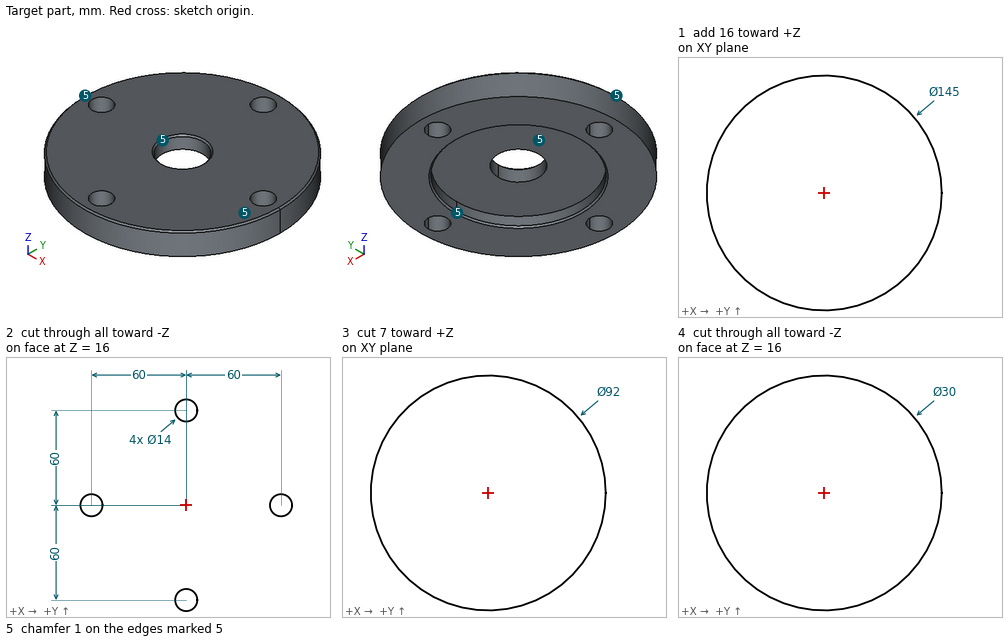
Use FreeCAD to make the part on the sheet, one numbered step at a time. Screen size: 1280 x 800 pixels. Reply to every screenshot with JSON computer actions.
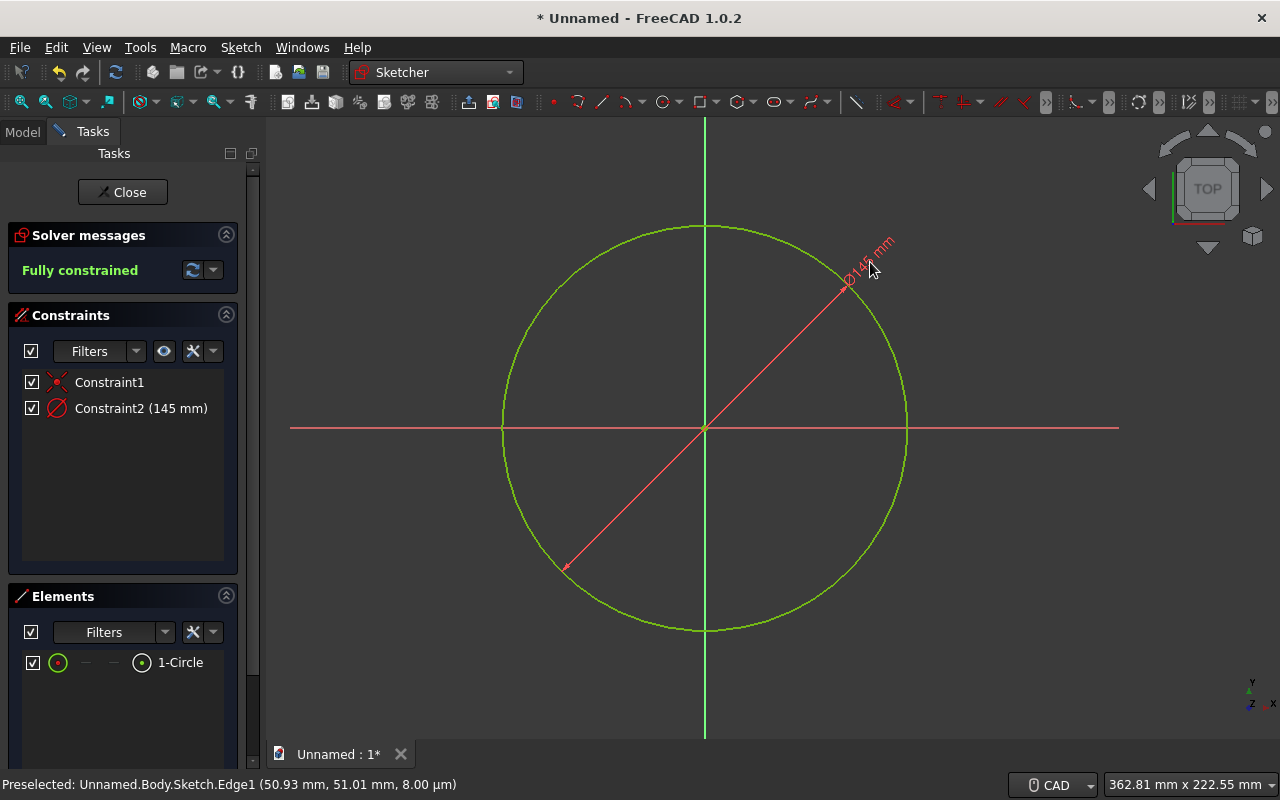
{"action": "left_click", "coordinate": [123, 192]}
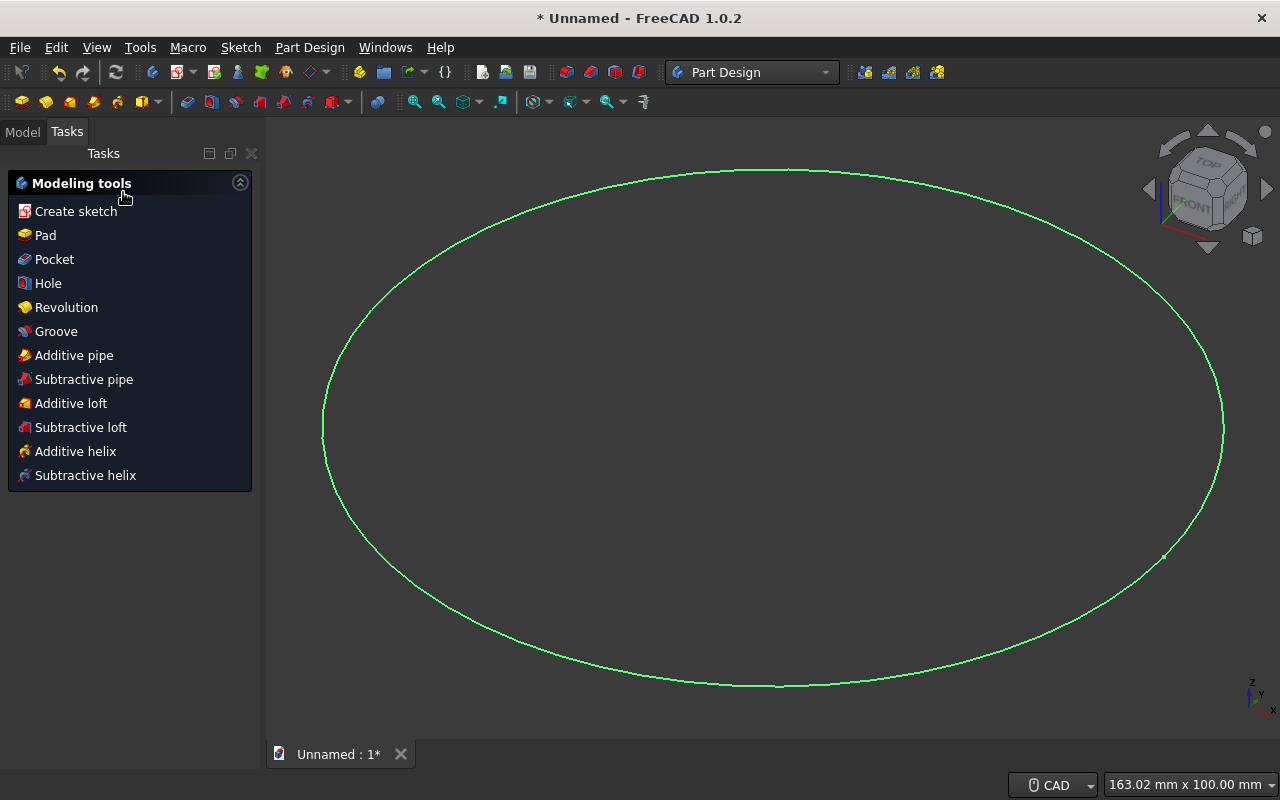
{"action": "left_click", "coordinate": [22, 102]}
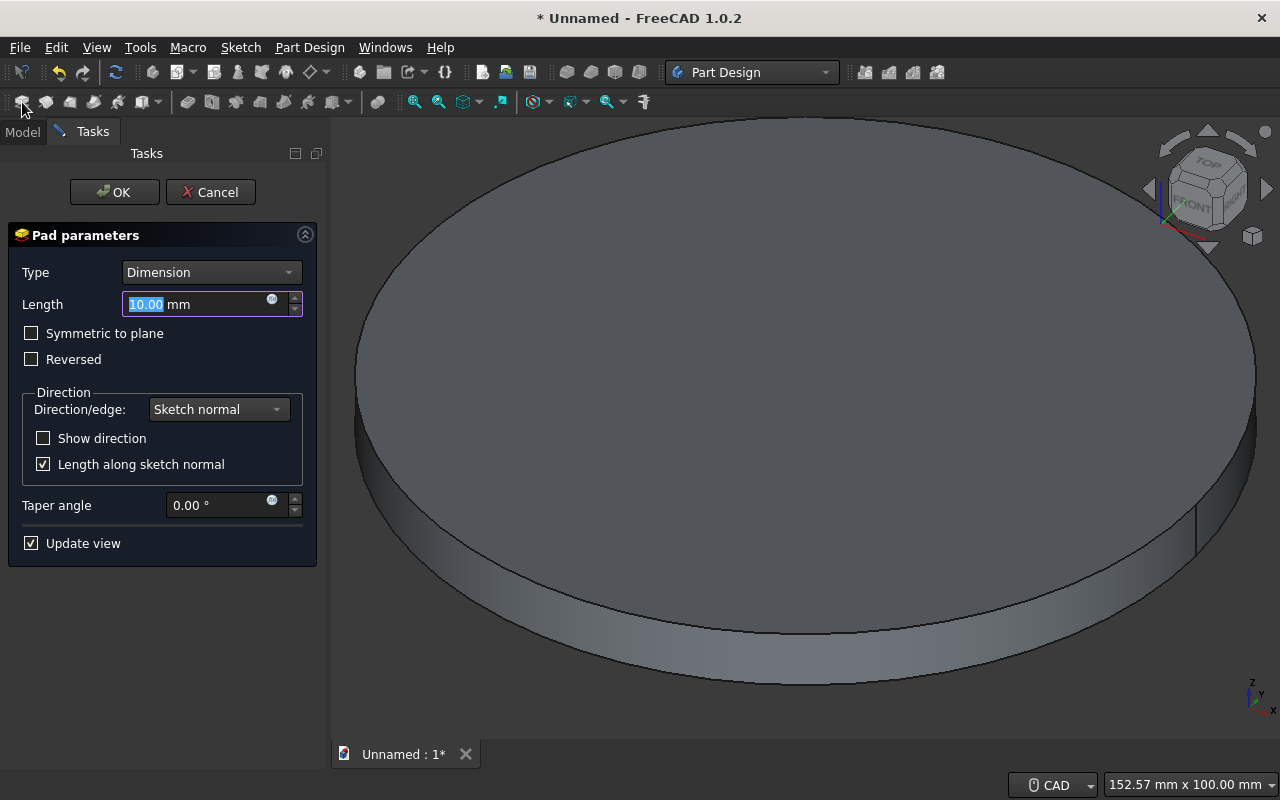
{"action": "type", "text": "16"}
{"action": "key", "text": "Tab"}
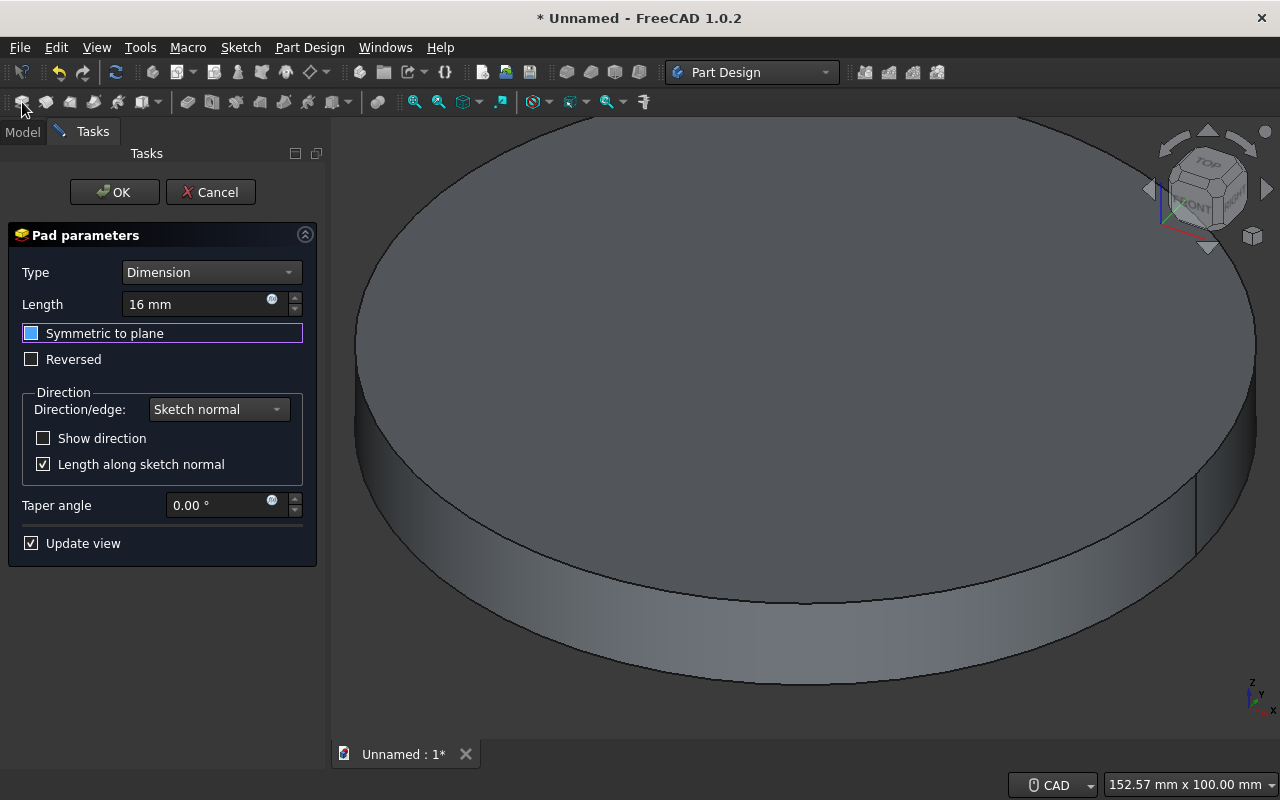
{"action": "left_click", "coordinate": [115, 192]}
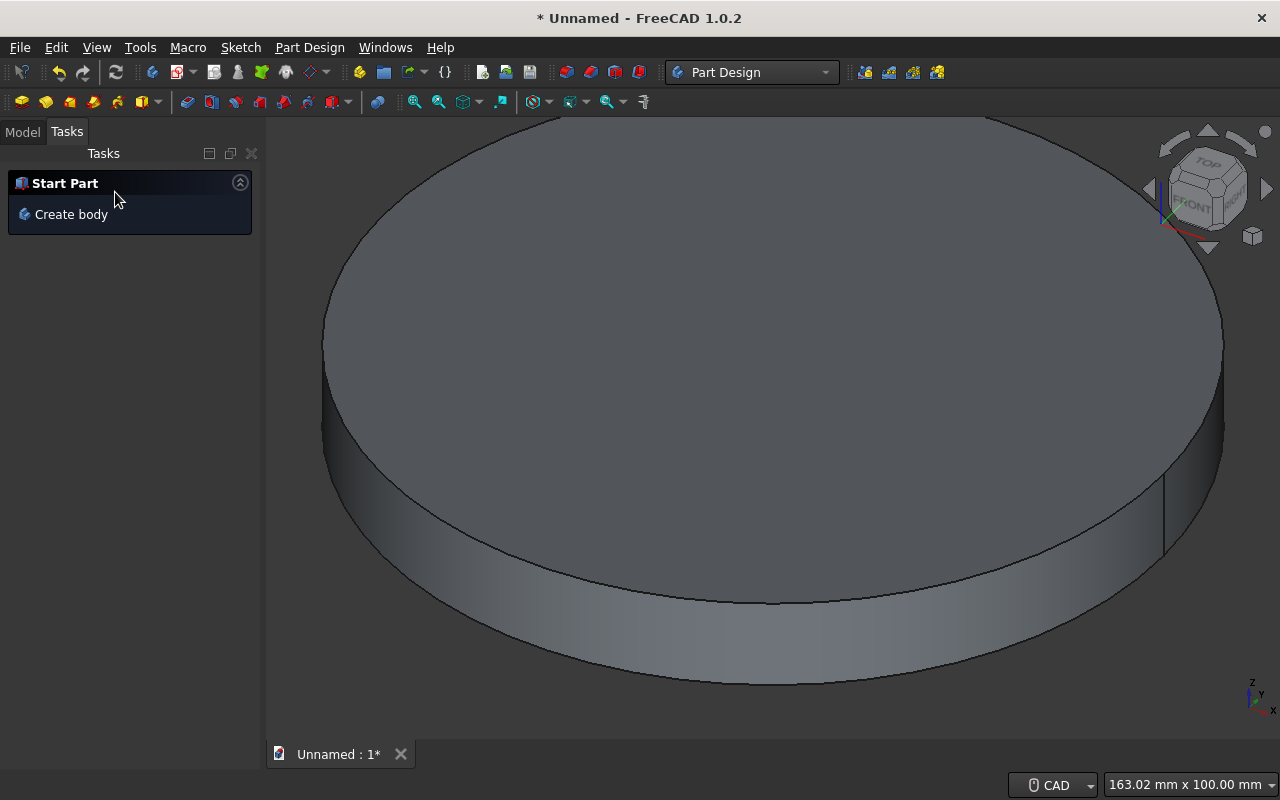
{"action": "key", "text": "v f"}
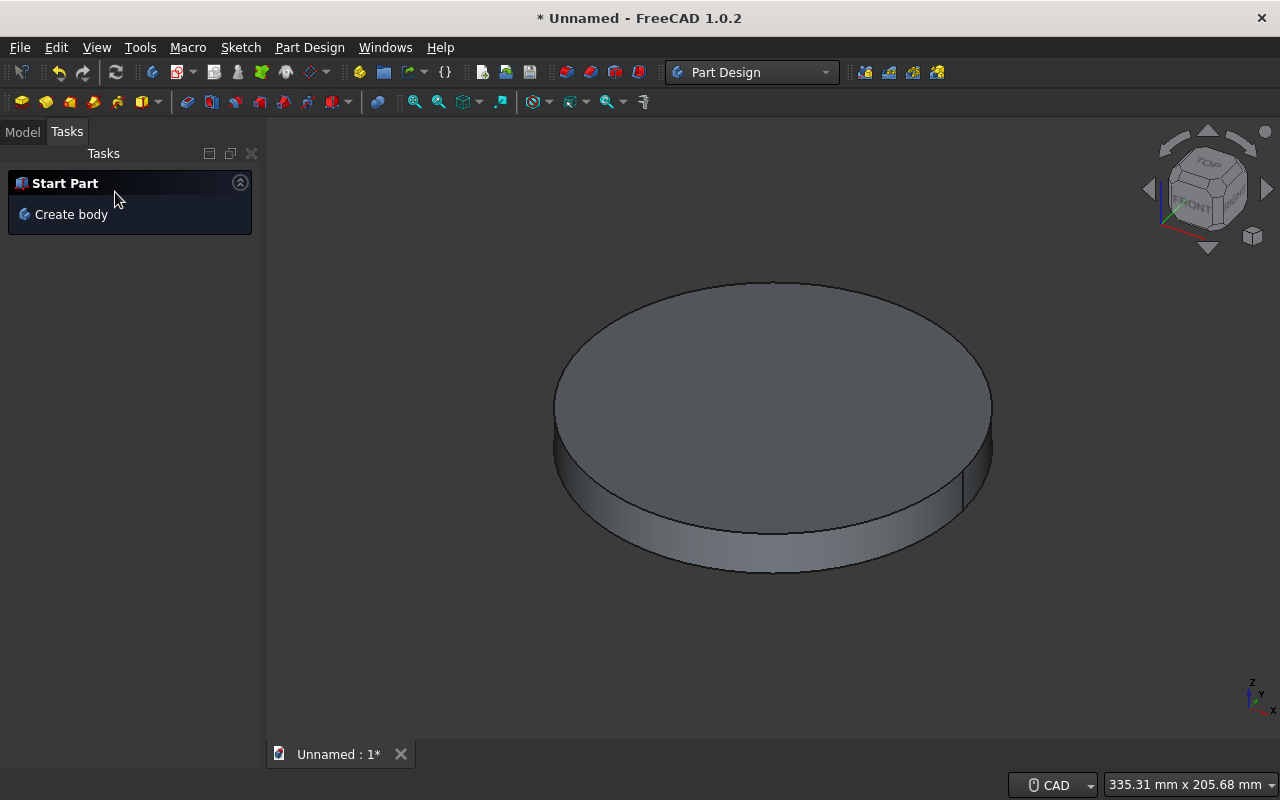
{"action": "left_click", "coordinate": [773, 407]}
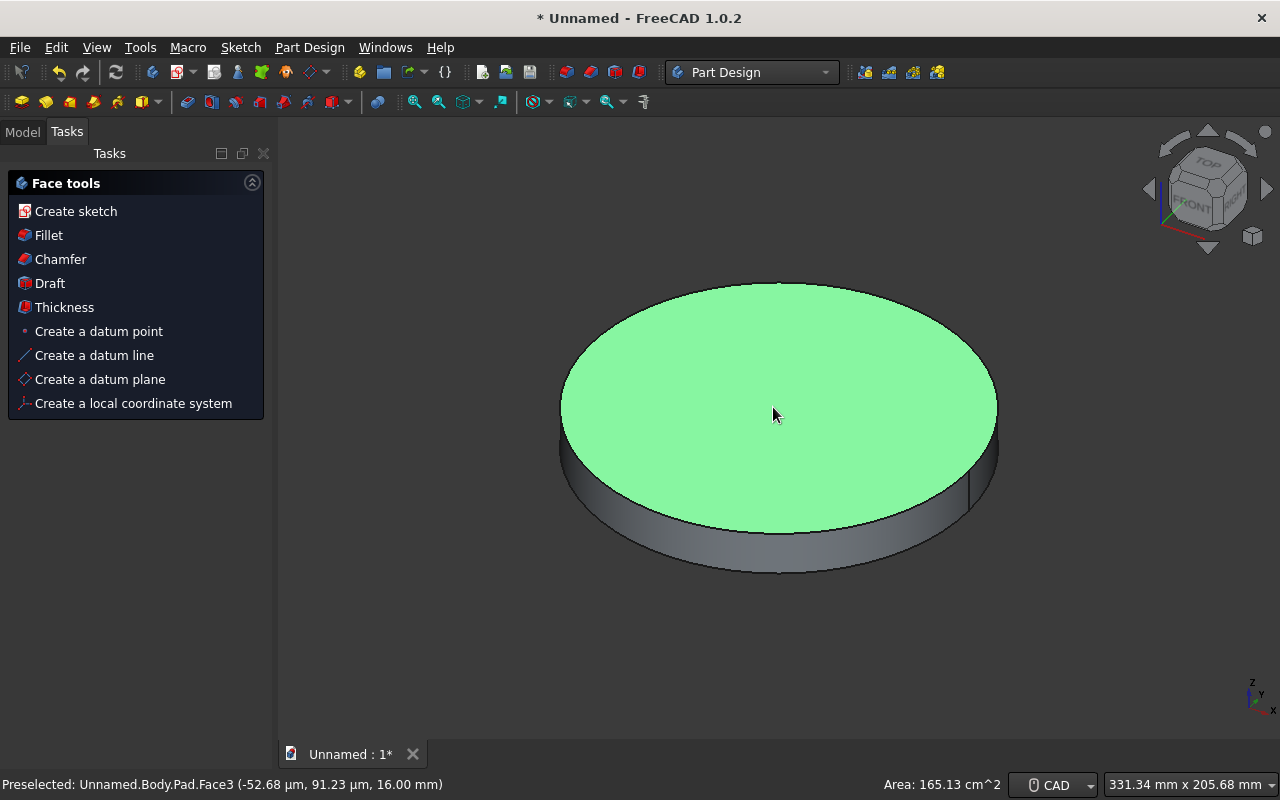
{"action": "left_click", "coordinate": [178, 72]}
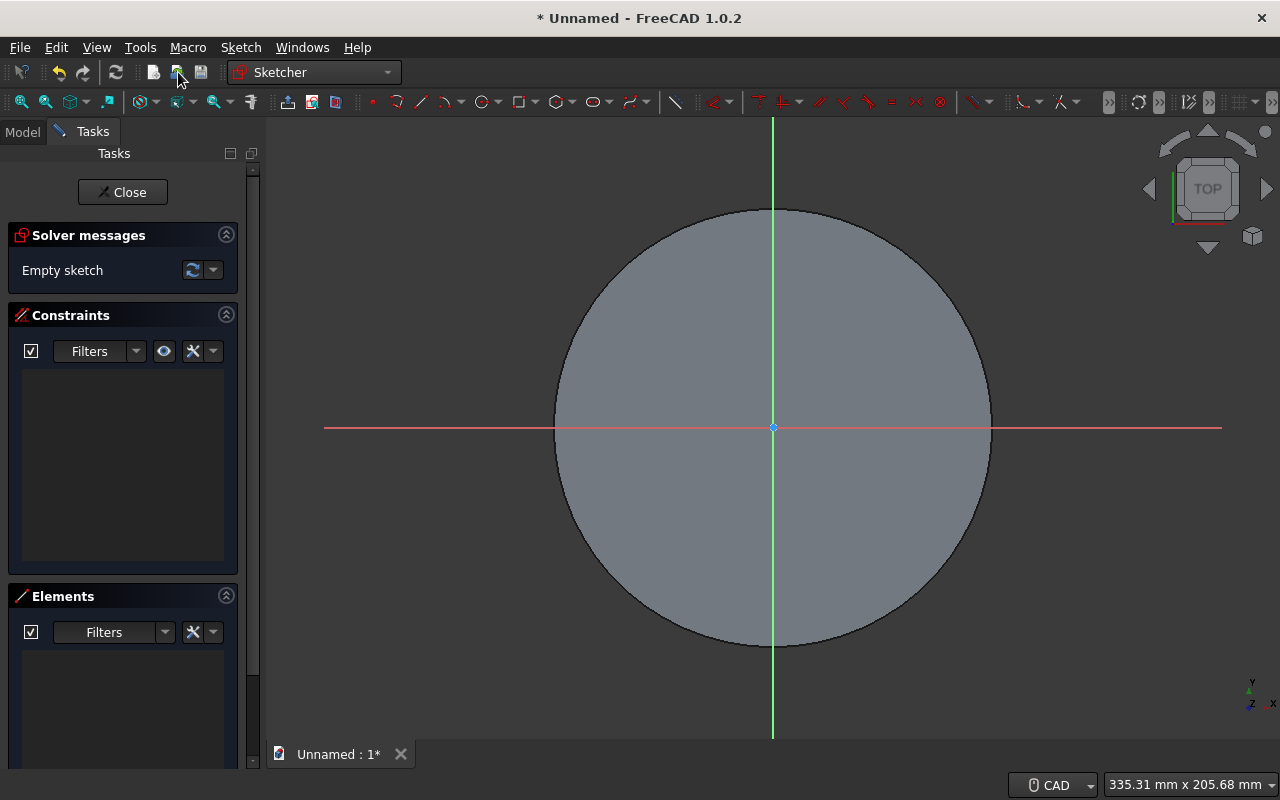
{"action": "key", "text": "g c"}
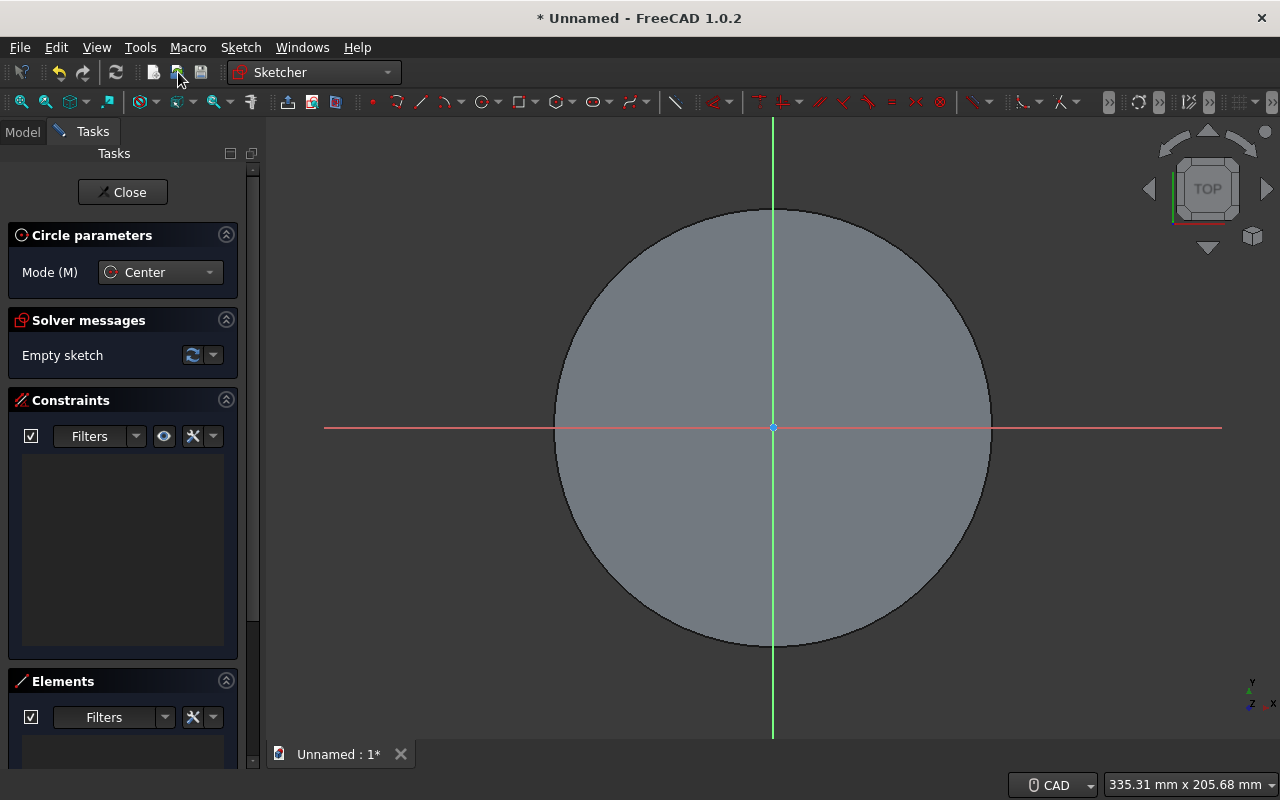
{"action": "left_click", "coordinate": [773, 247]}
{"action": "left_click", "coordinate": [788, 232]}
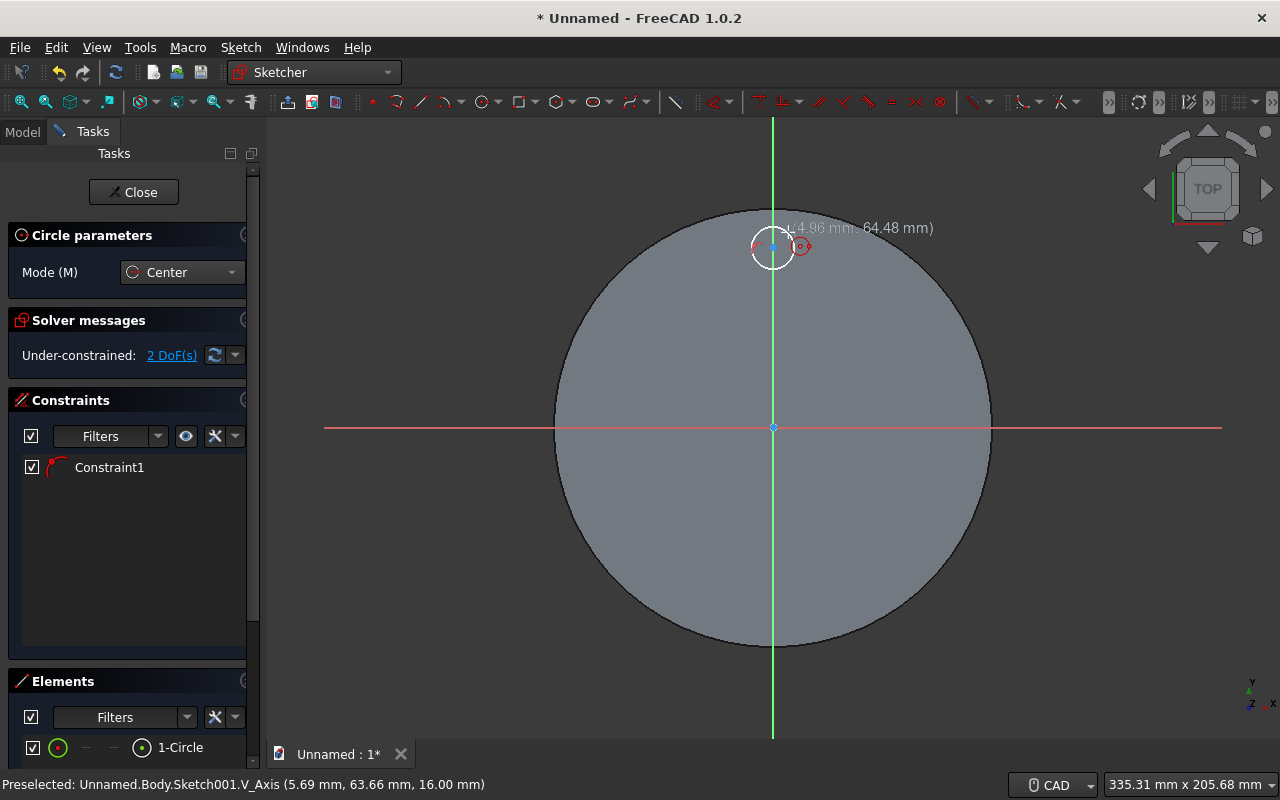
{"action": "left_click", "coordinate": [954, 428]}
{"action": "left_click", "coordinate": [969, 413]}